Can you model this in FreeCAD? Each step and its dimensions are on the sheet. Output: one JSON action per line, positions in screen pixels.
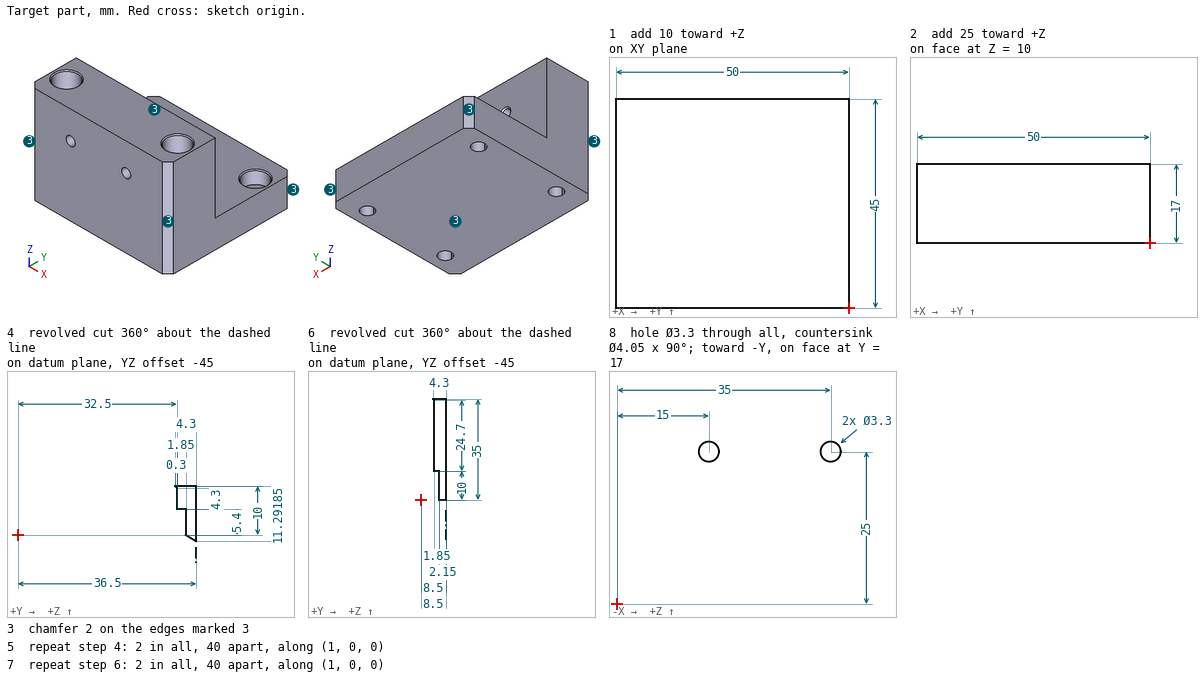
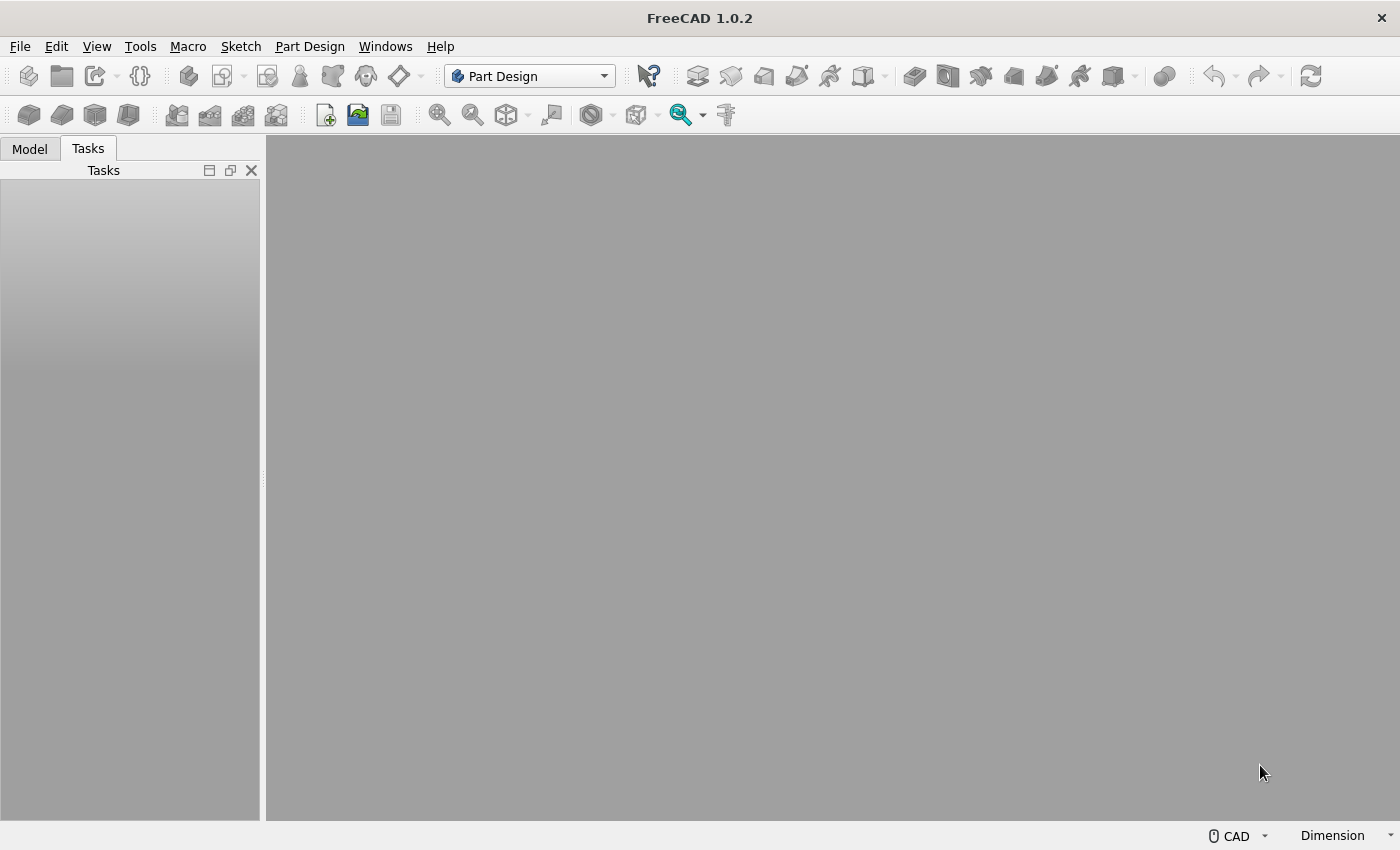
{"action": "key", "text": "ctrl+n"}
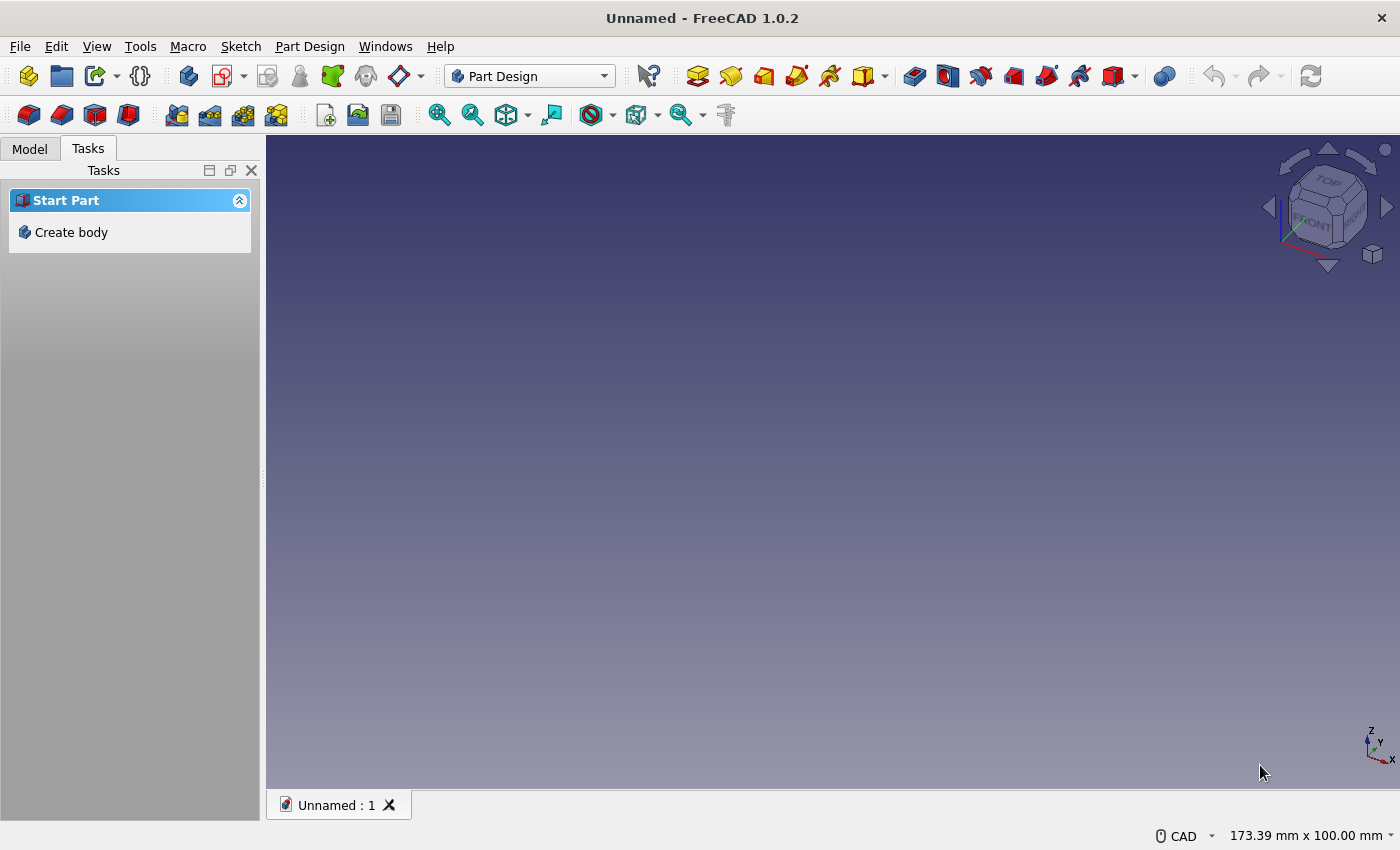
{"action": "left_click", "coordinate": [222, 76]}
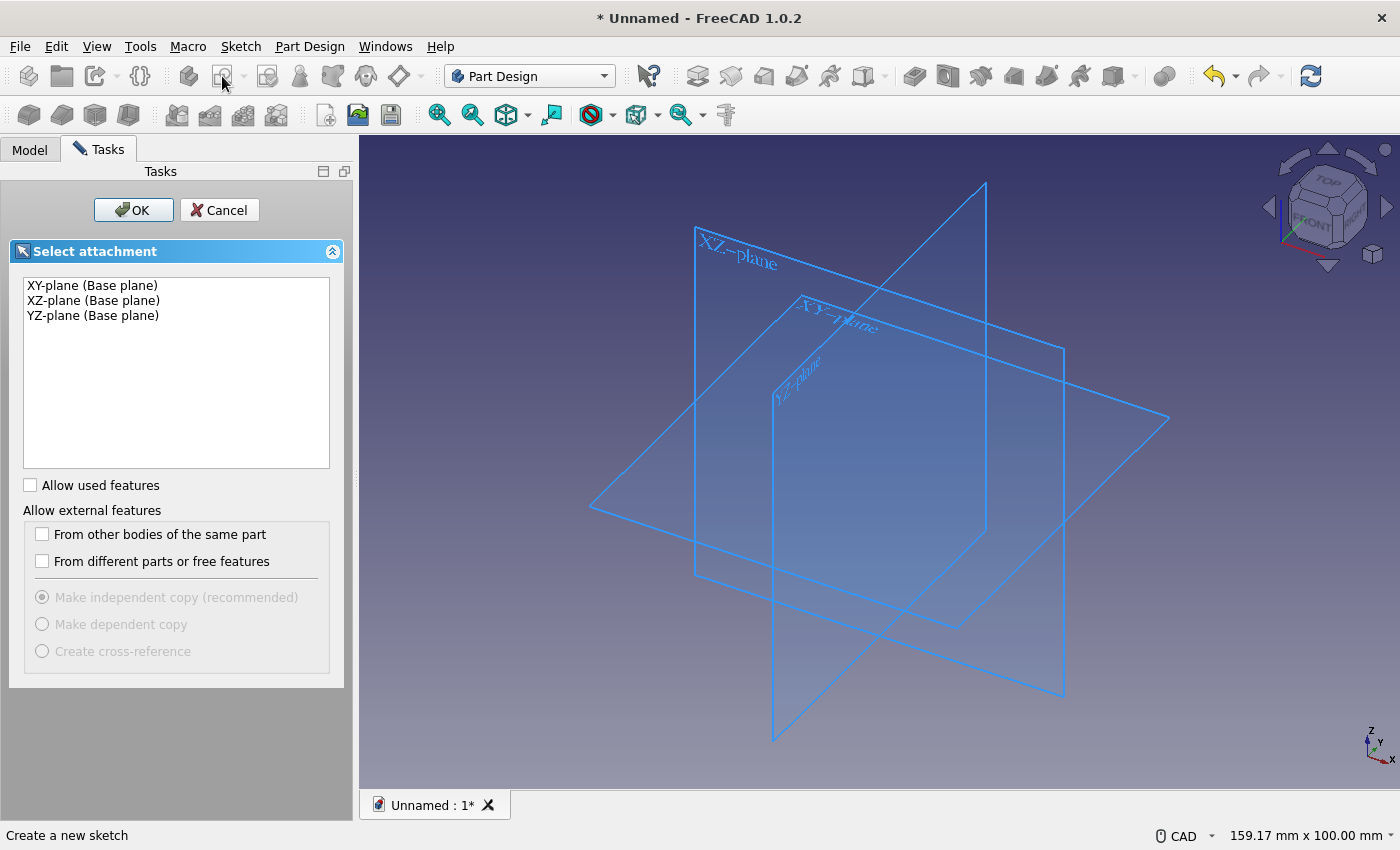
{"action": "left_click", "coordinate": [84, 286]}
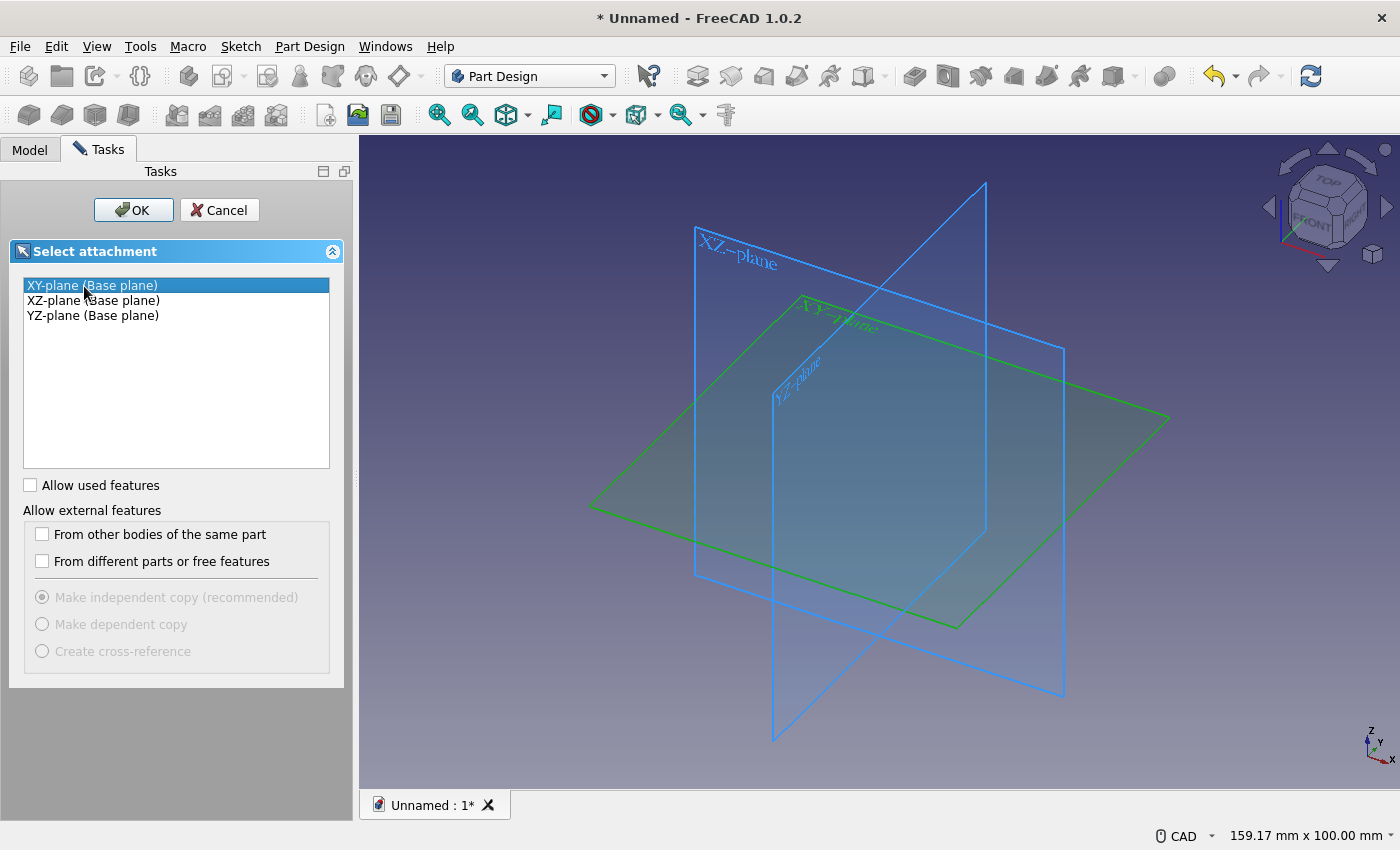
{"action": "left_click", "coordinate": [134, 210]}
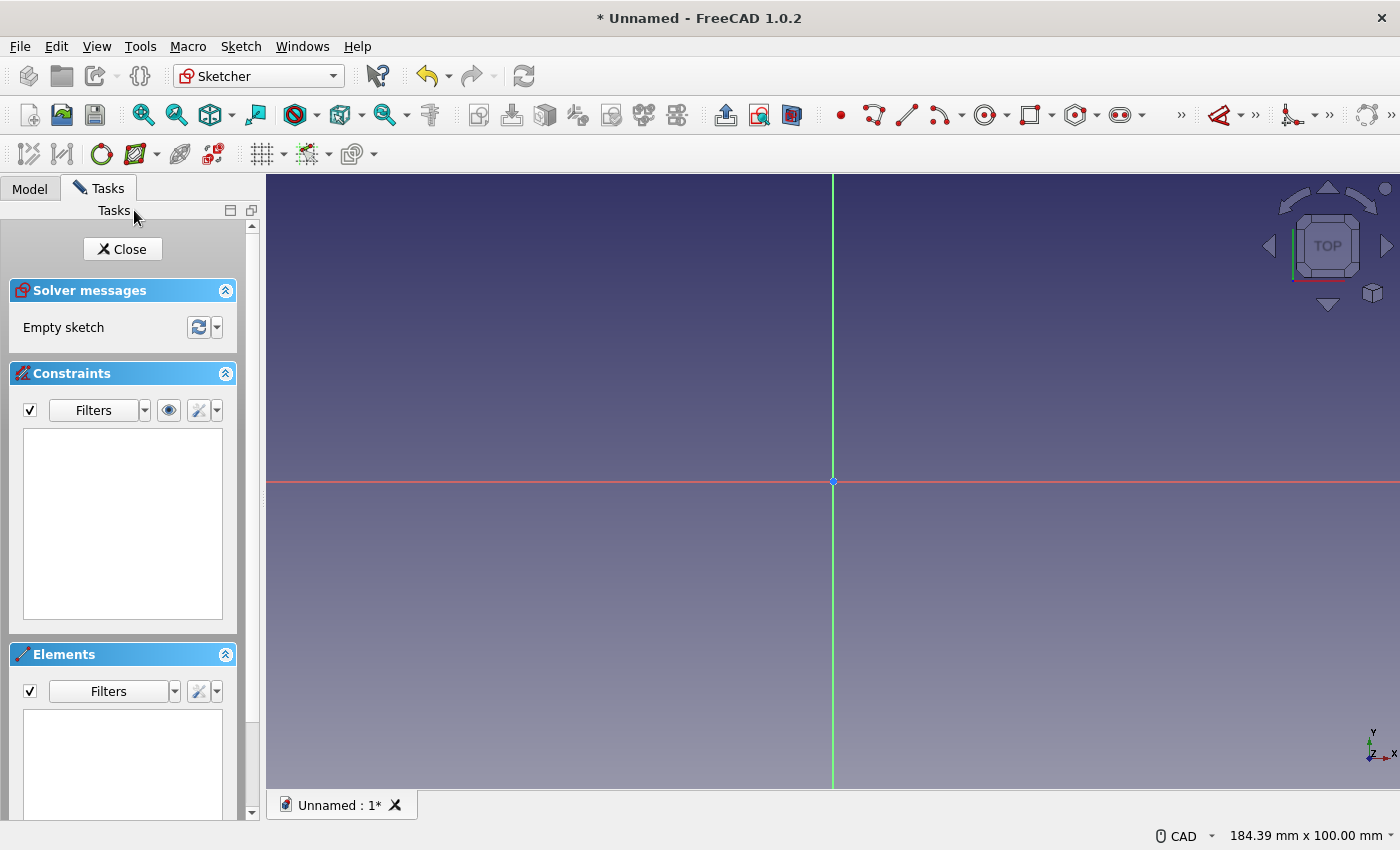
{"action": "scroll", "coordinate": [1150, 761], "scroll_direction": "down", "scroll_amount": 1}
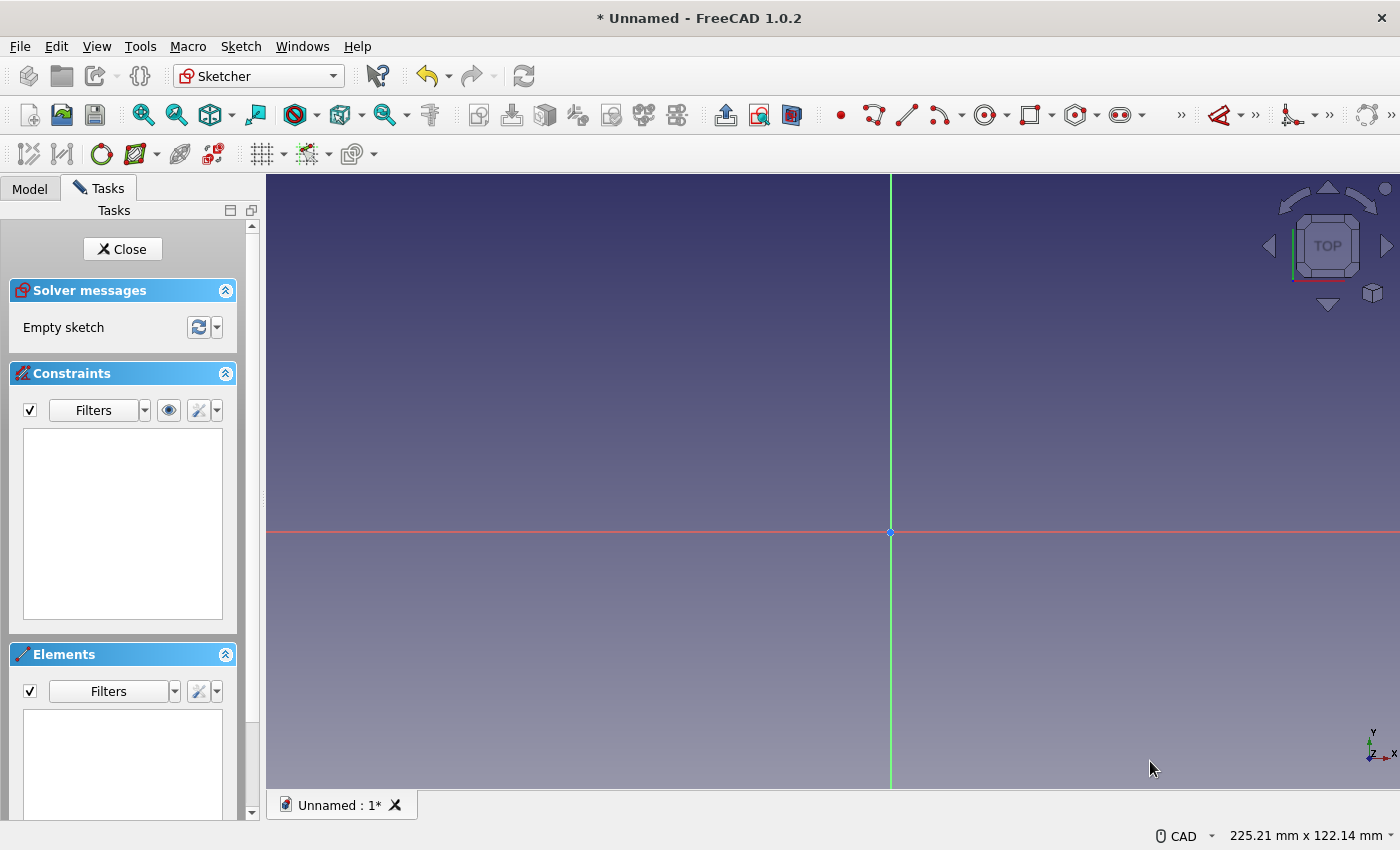
{"action": "scroll", "coordinate": [765, 343], "scroll_direction": "up", "scroll_amount": 3}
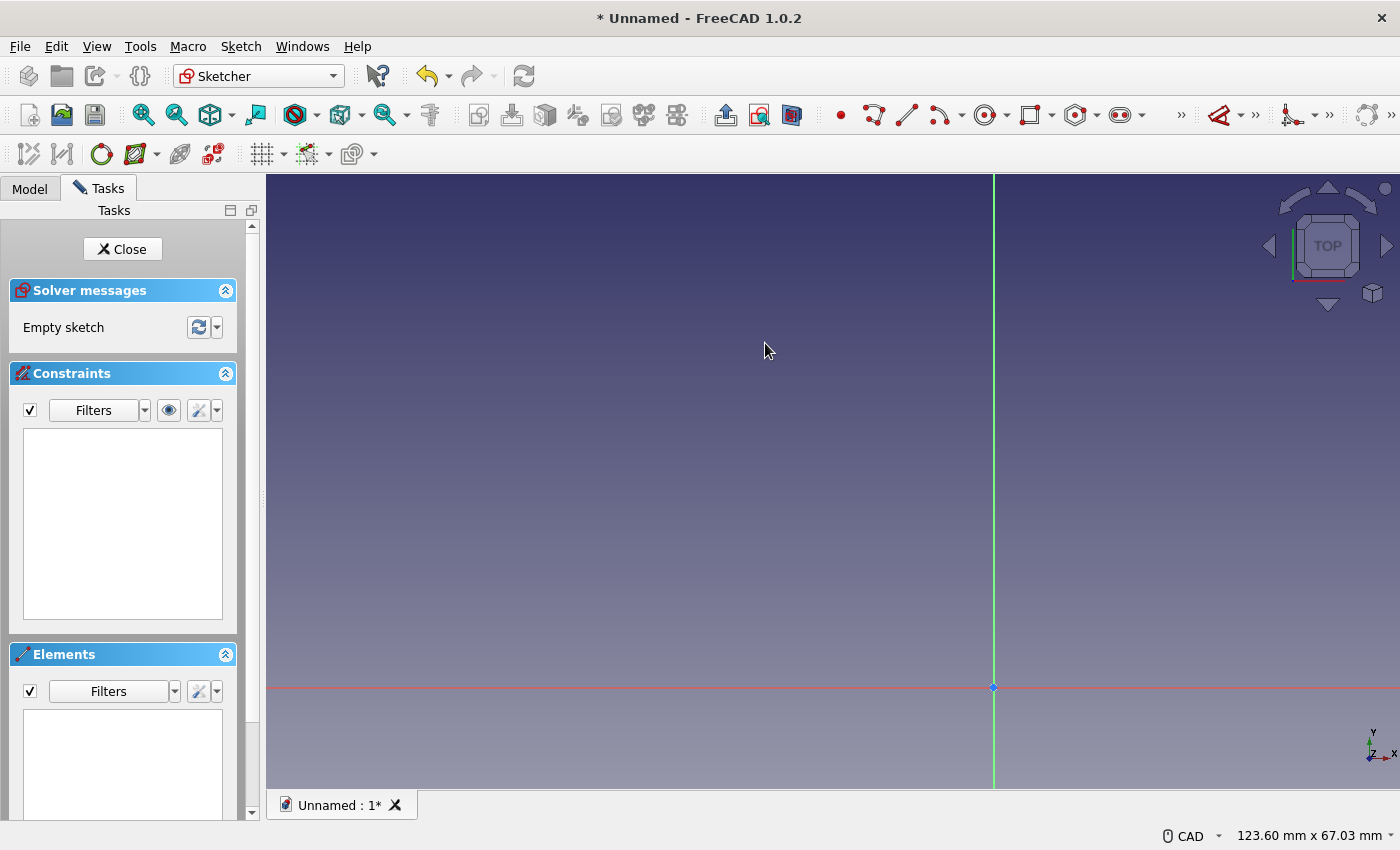
{"action": "key", "text": "g r"}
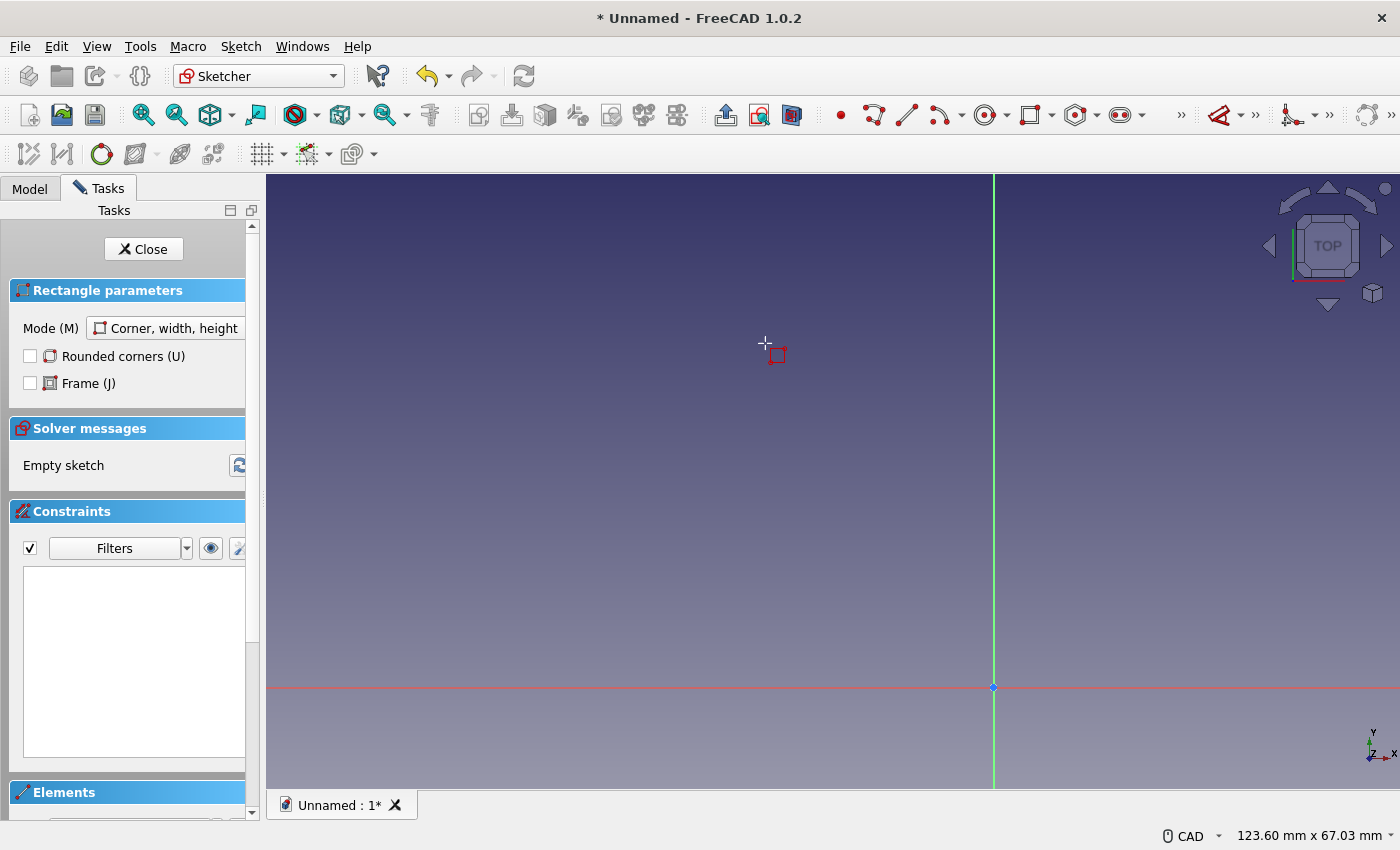
{"action": "left_click", "coordinate": [994, 688]}
{"action": "left_click", "coordinate": [535, 275]}
{"action": "key", "text": "Escape"}